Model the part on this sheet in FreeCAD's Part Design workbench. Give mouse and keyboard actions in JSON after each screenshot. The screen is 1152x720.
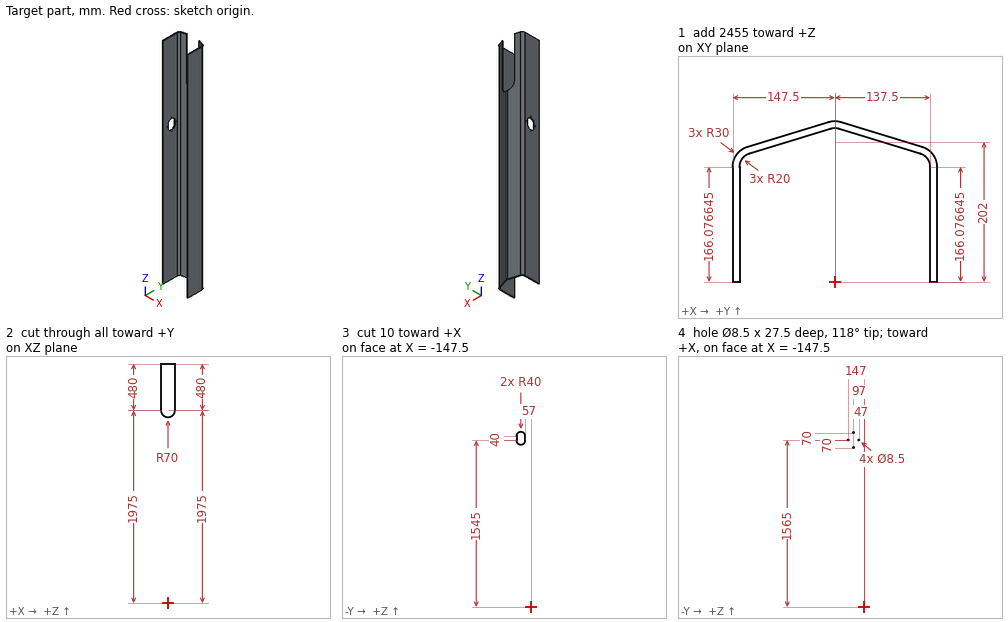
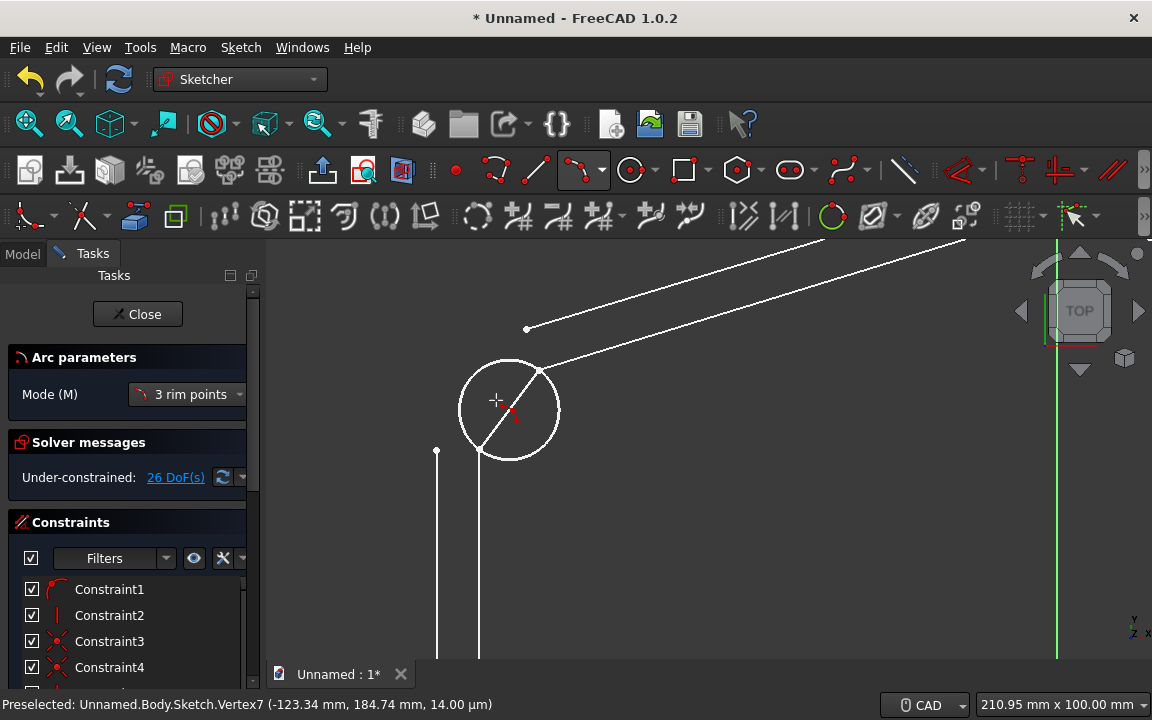
{"action": "left_click", "coordinate": [496, 398]}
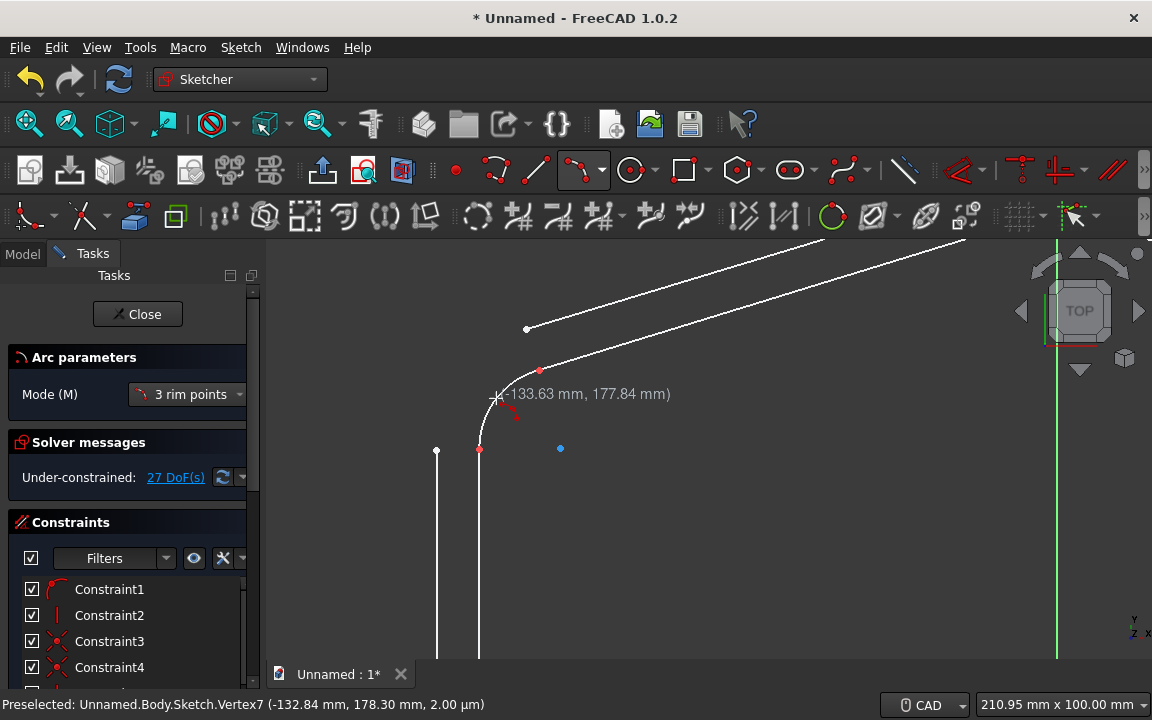
{"action": "scroll", "coordinate": [504, 380], "scroll_direction": "down", "scroll_amount": 7}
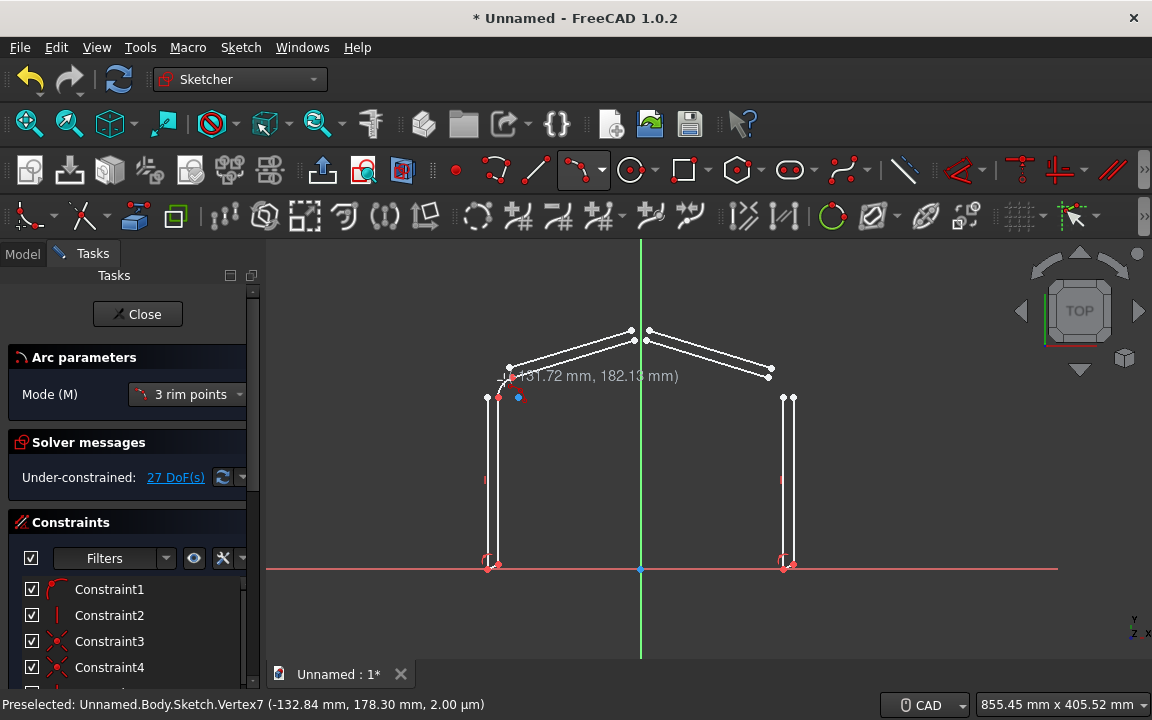
{"action": "scroll", "coordinate": [635, 340], "scroll_direction": "up", "scroll_amount": 5}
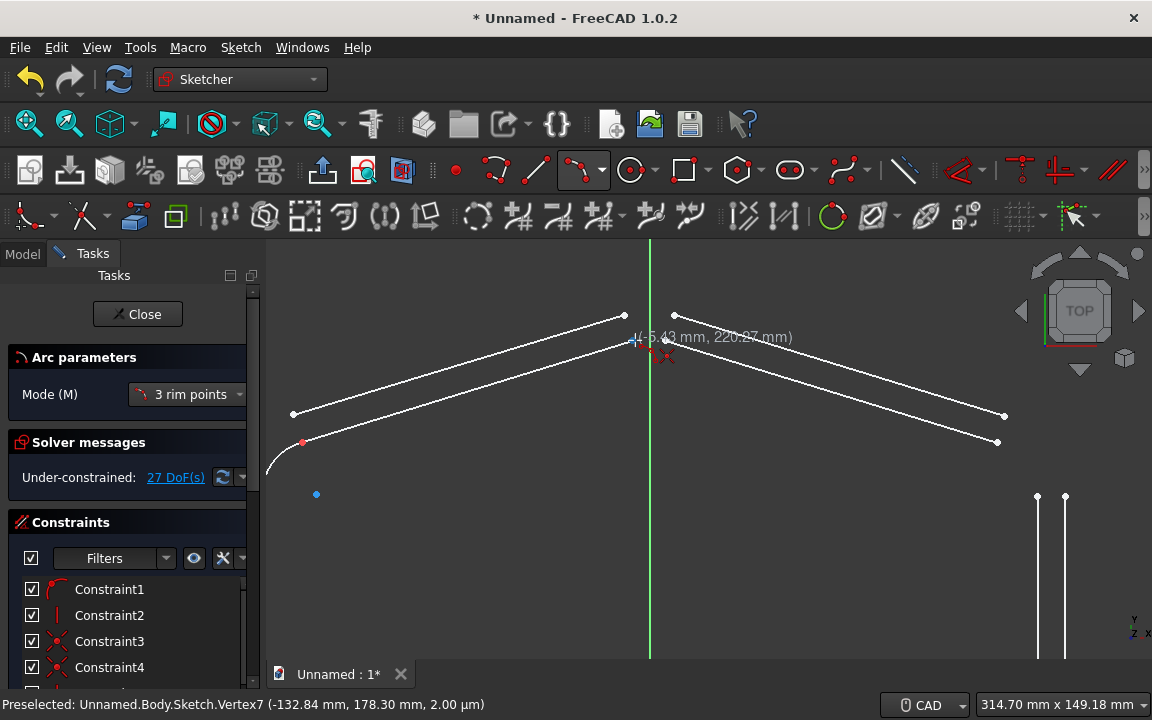
{"action": "left_click", "coordinate": [633, 341]}
{"action": "left_click", "coordinate": [666, 341]}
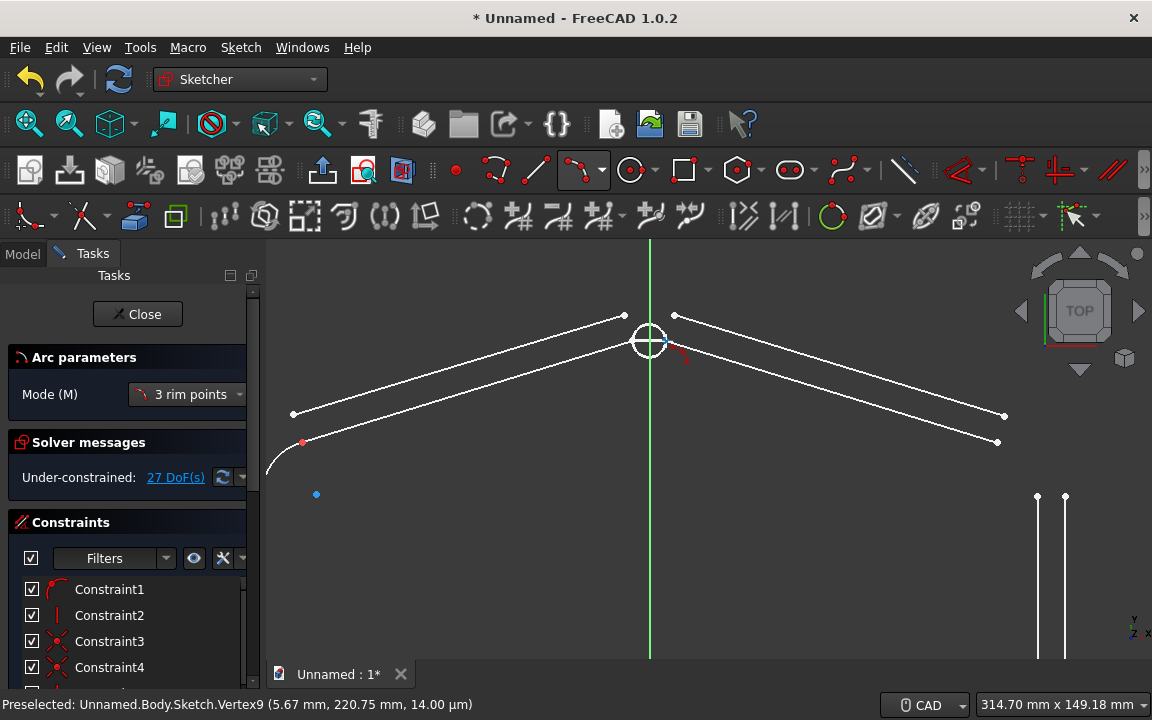
{"action": "scroll", "coordinate": [653, 338], "scroll_direction": "up", "scroll_amount": 10}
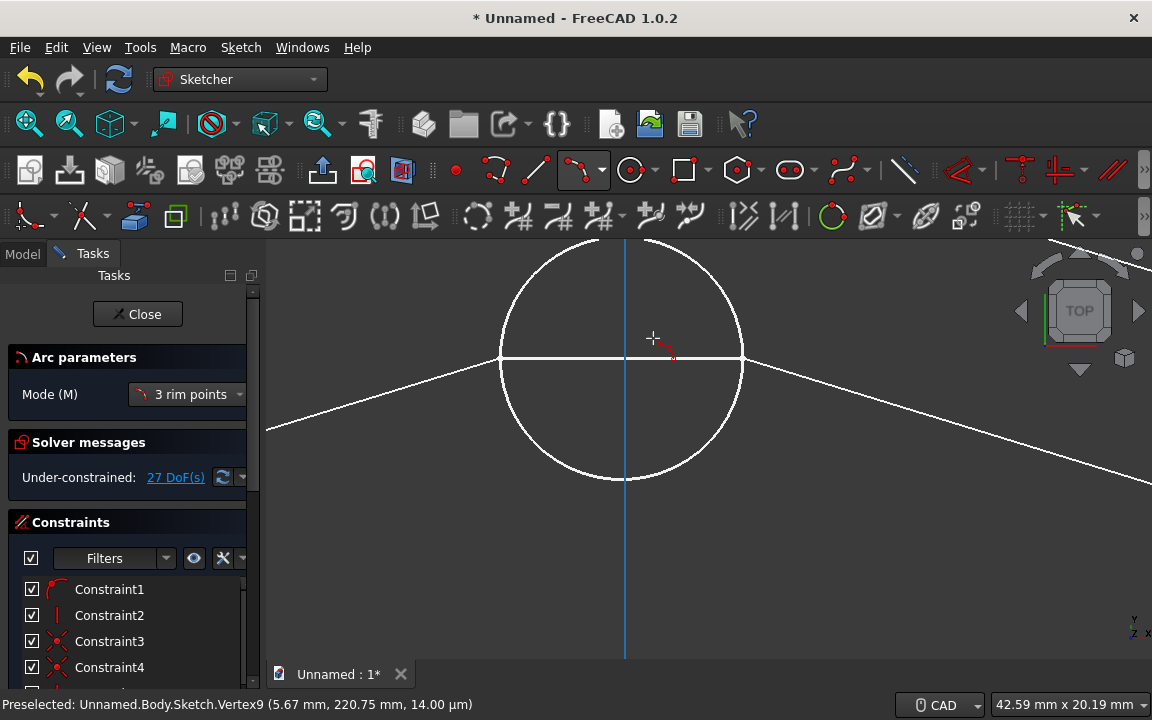
{"action": "left_click", "coordinate": [650, 333]}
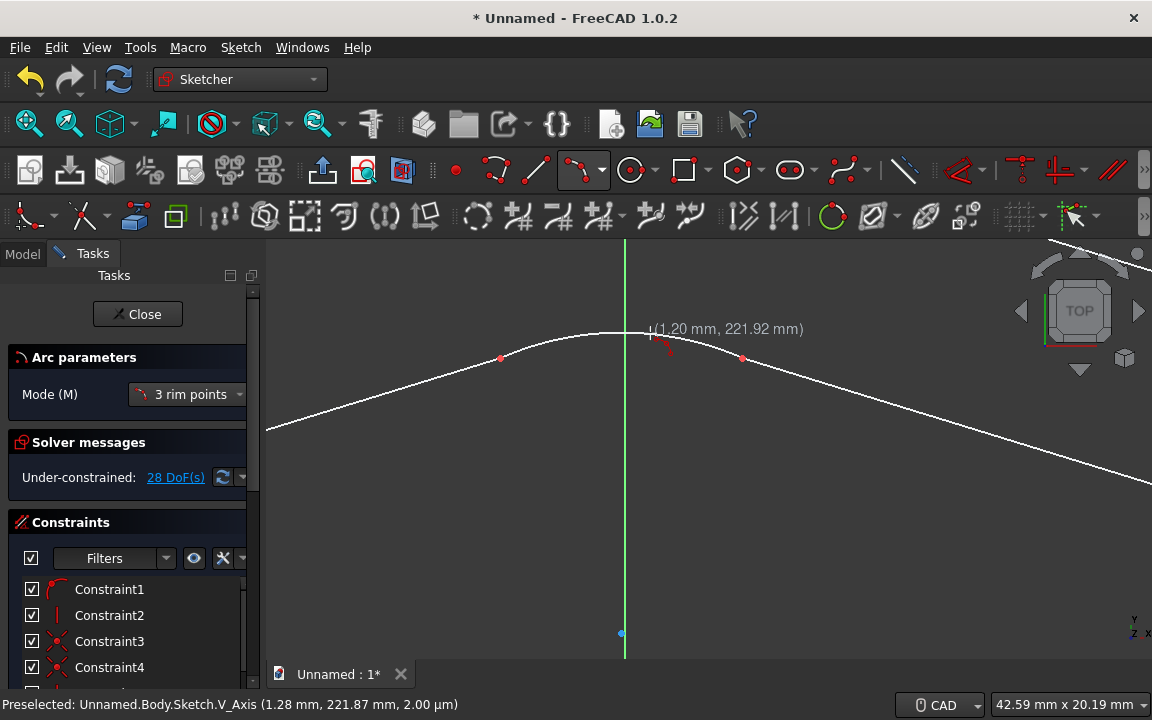
{"action": "scroll", "coordinate": [641, 340], "scroll_direction": "down", "scroll_amount": 15}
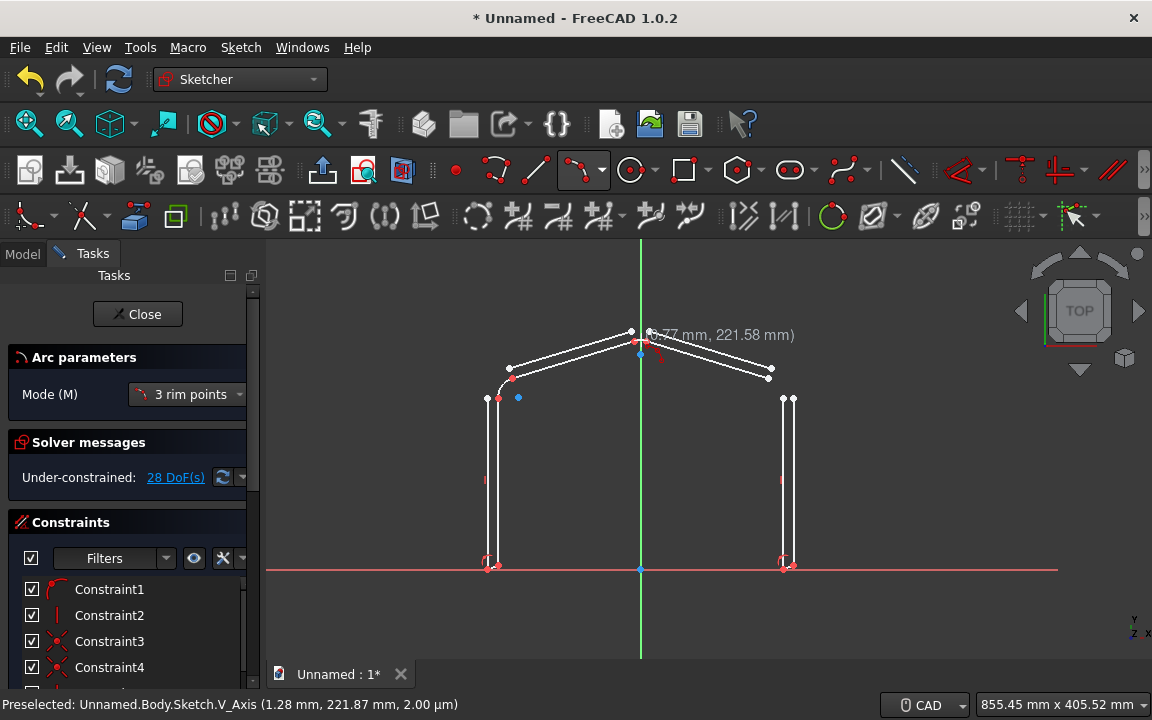
{"action": "scroll", "coordinate": [768, 378], "scroll_direction": "up", "scroll_amount": 3}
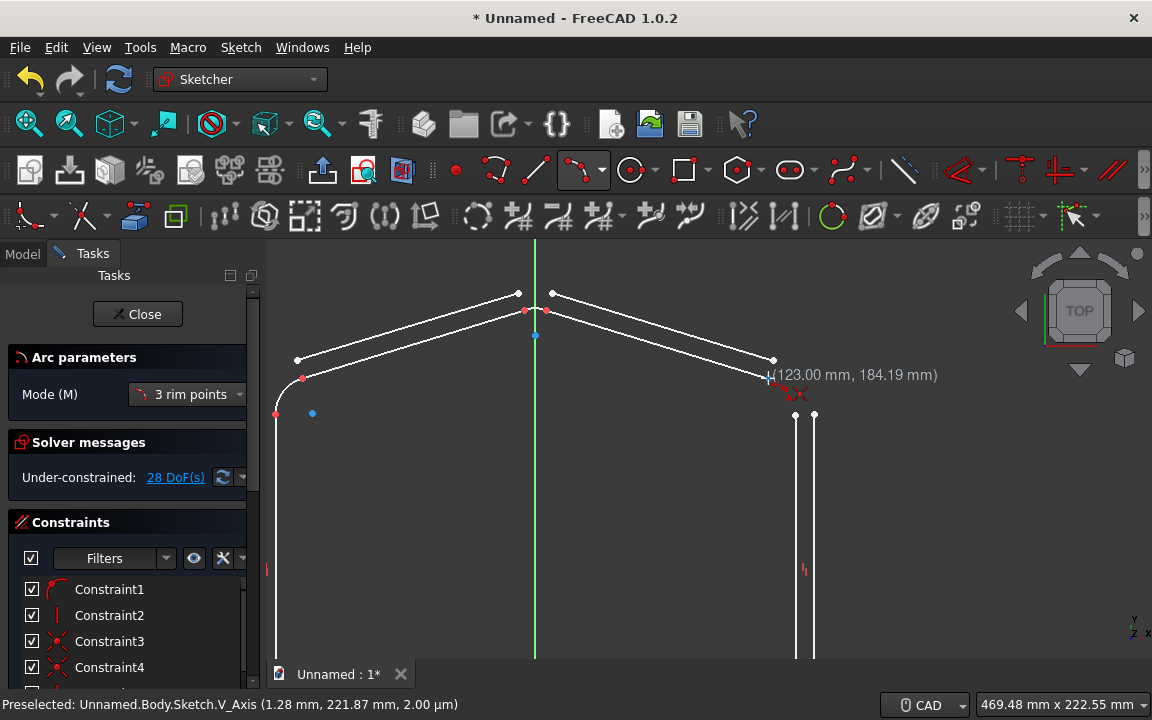
{"action": "left_click", "coordinate": [768, 379]}
{"action": "left_click", "coordinate": [796, 415]}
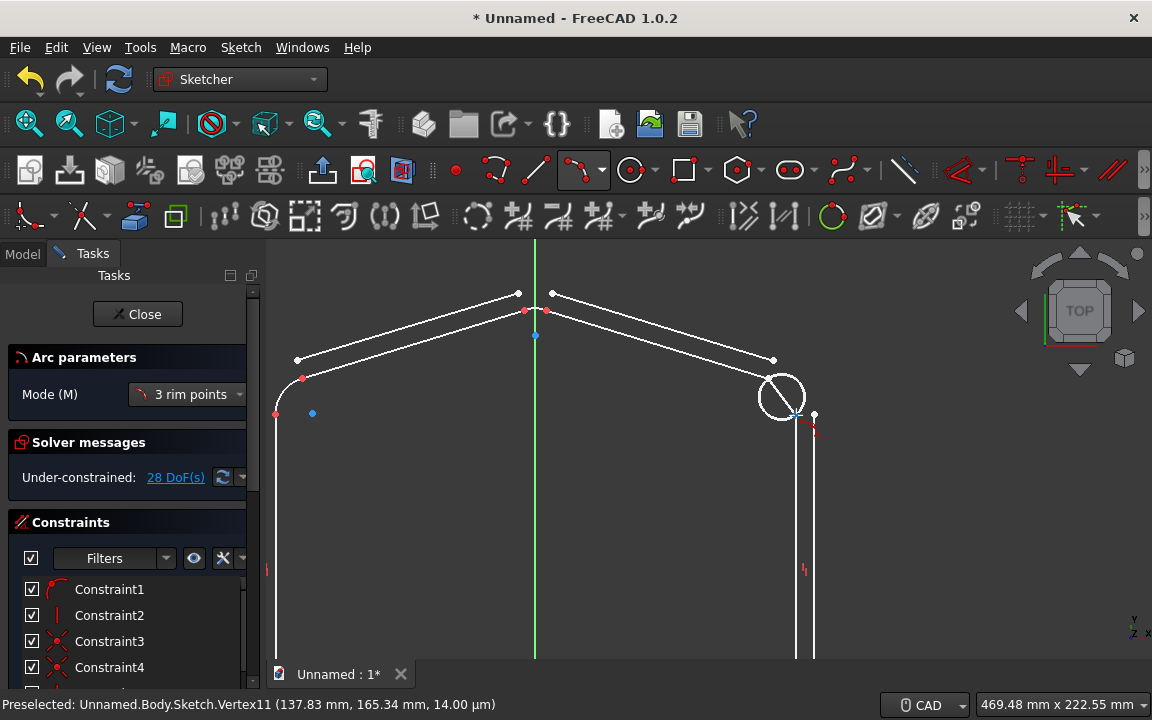
{"action": "scroll", "coordinate": [787, 391], "scroll_direction": "up", "scroll_amount": 4}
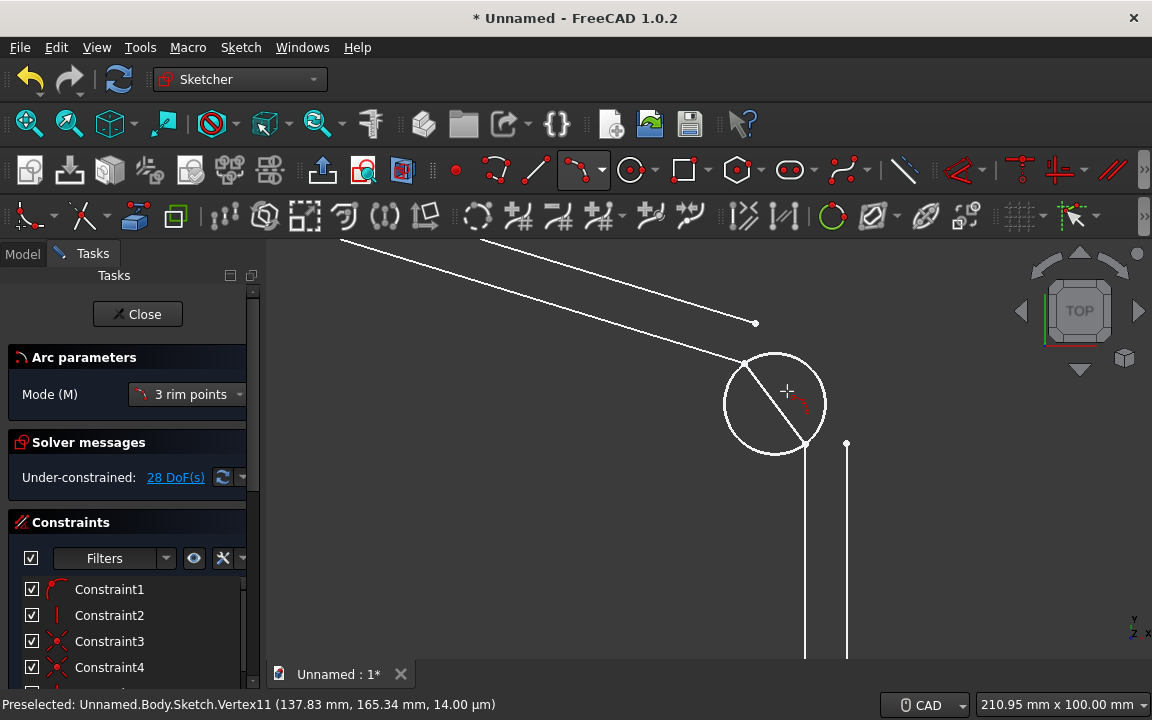
{"action": "left_click", "coordinate": [787, 391]}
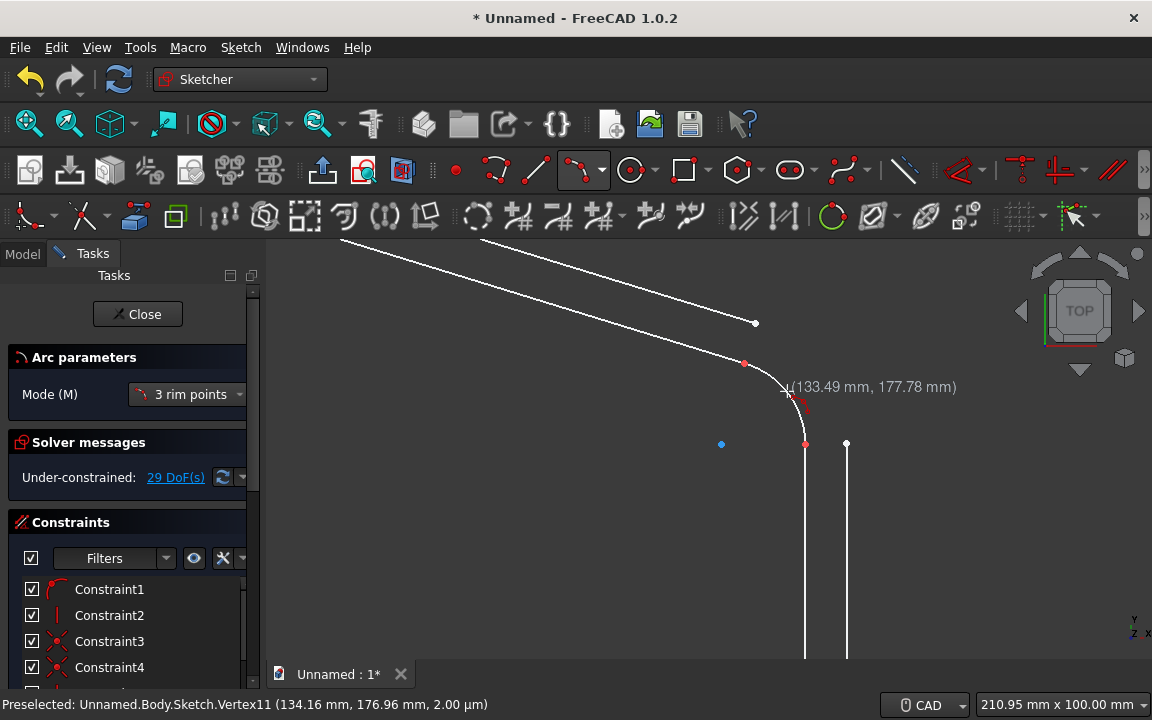
{"action": "left_click", "coordinate": [847, 443]}
{"action": "left_click", "coordinate": [756, 324]}
{"action": "left_click", "coordinate": [821, 366]}